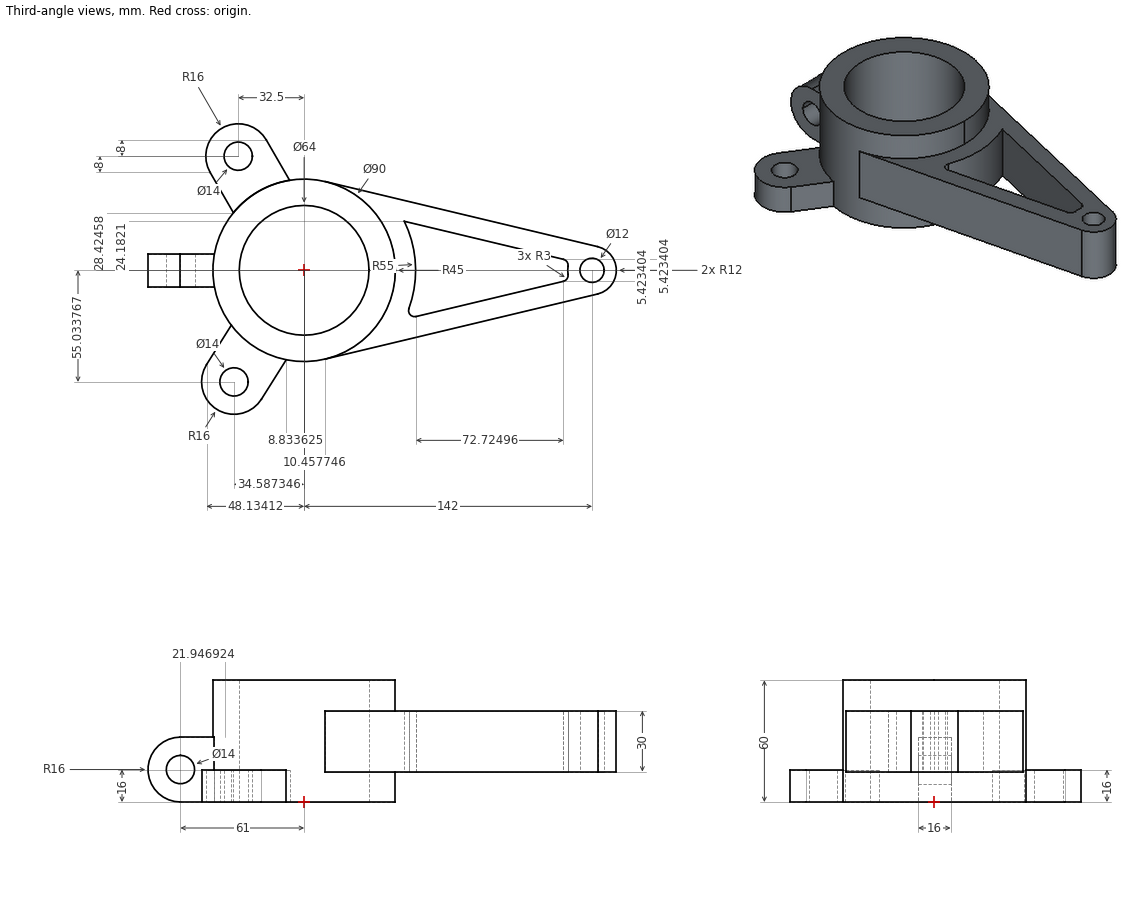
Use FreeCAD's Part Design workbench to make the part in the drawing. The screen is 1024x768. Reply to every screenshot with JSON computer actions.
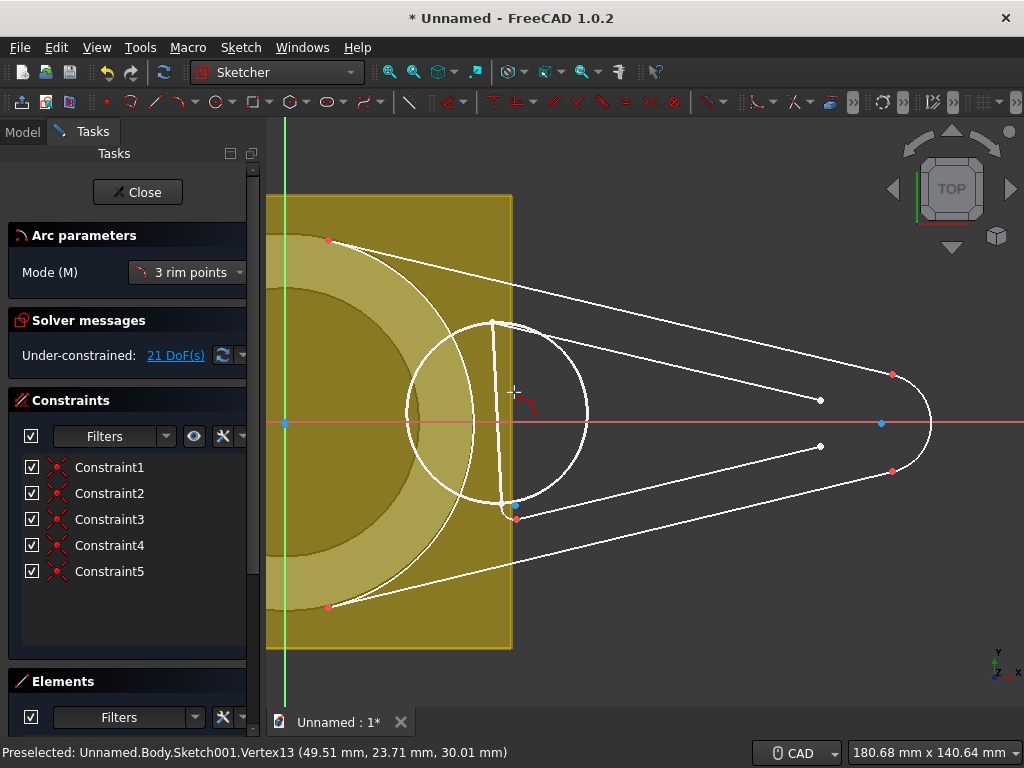
{"action": "left_click", "coordinate": [514, 392]}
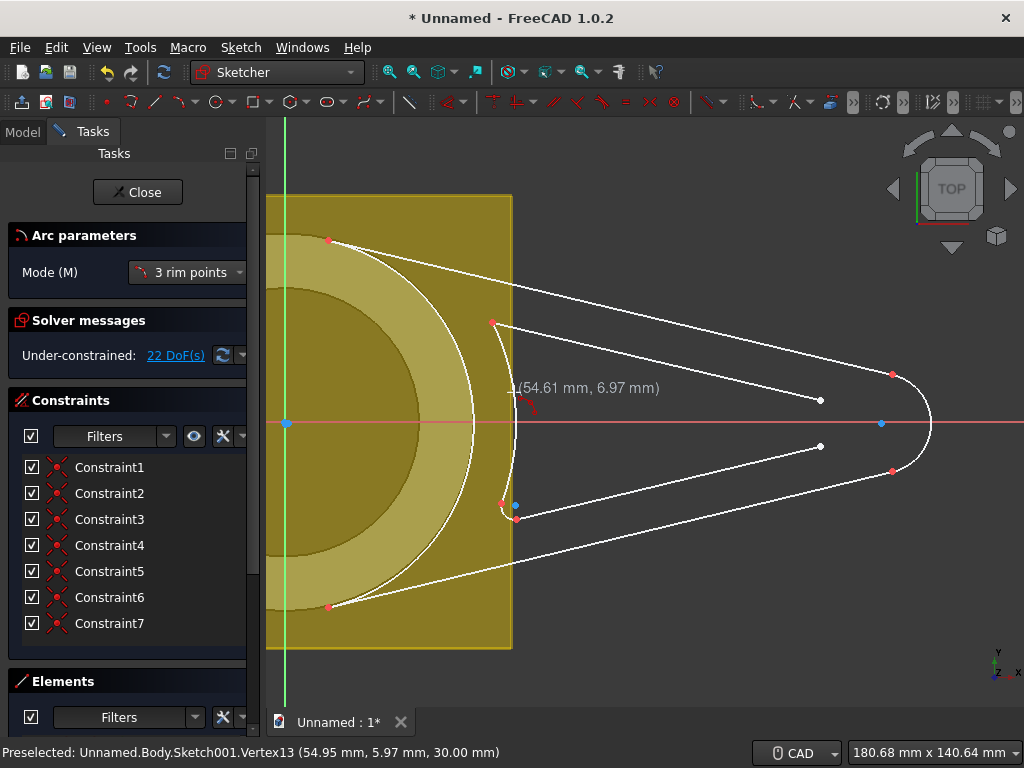
{"action": "left_click", "coordinate": [821, 400]}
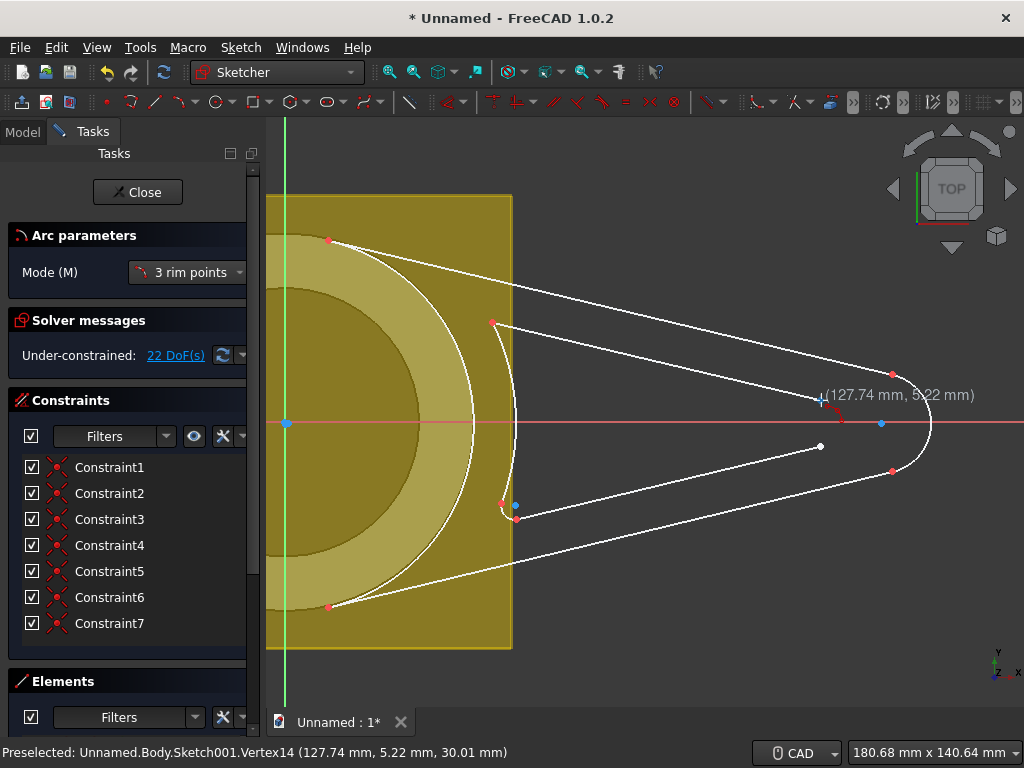
{"action": "scroll", "coordinate": [831, 414], "scroll_direction": "up", "scroll_amount": 4}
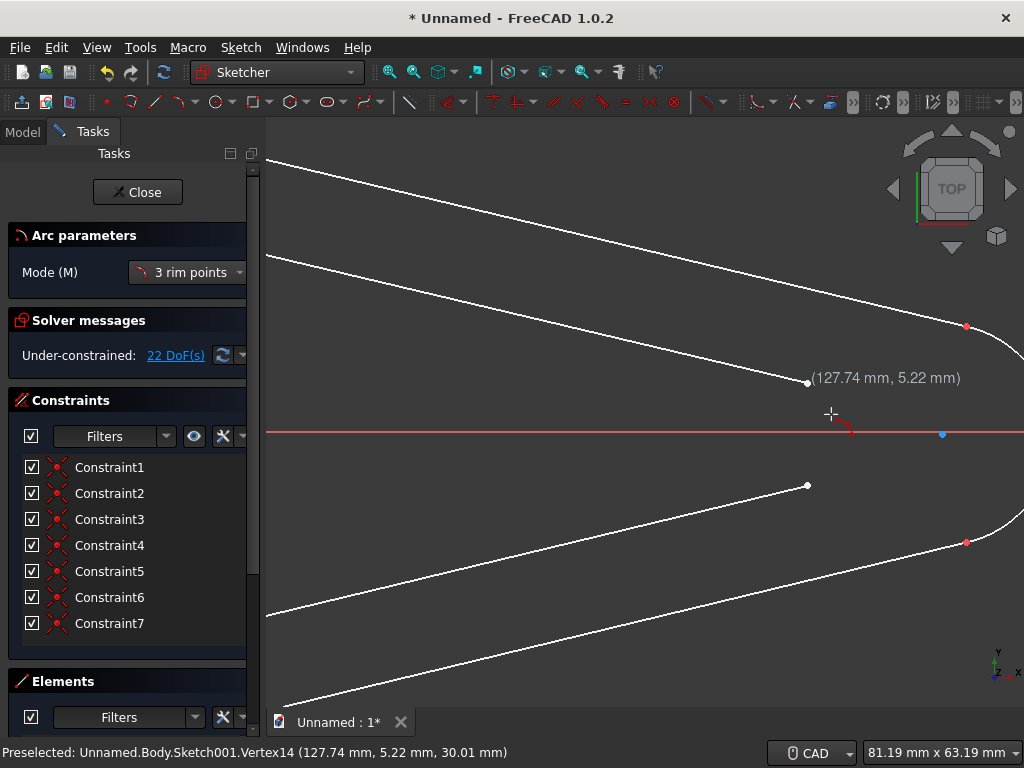
{"action": "left_click", "coordinate": [830, 413]}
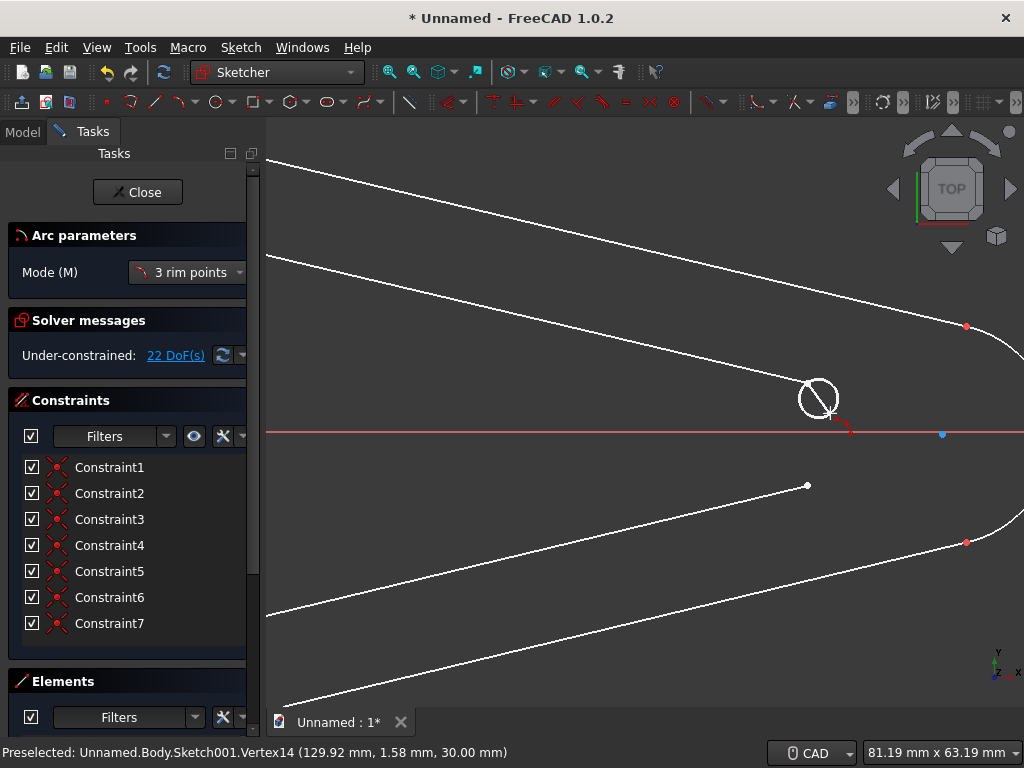
{"action": "scroll", "coordinate": [826, 393], "scroll_direction": "up", "scroll_amount": 4}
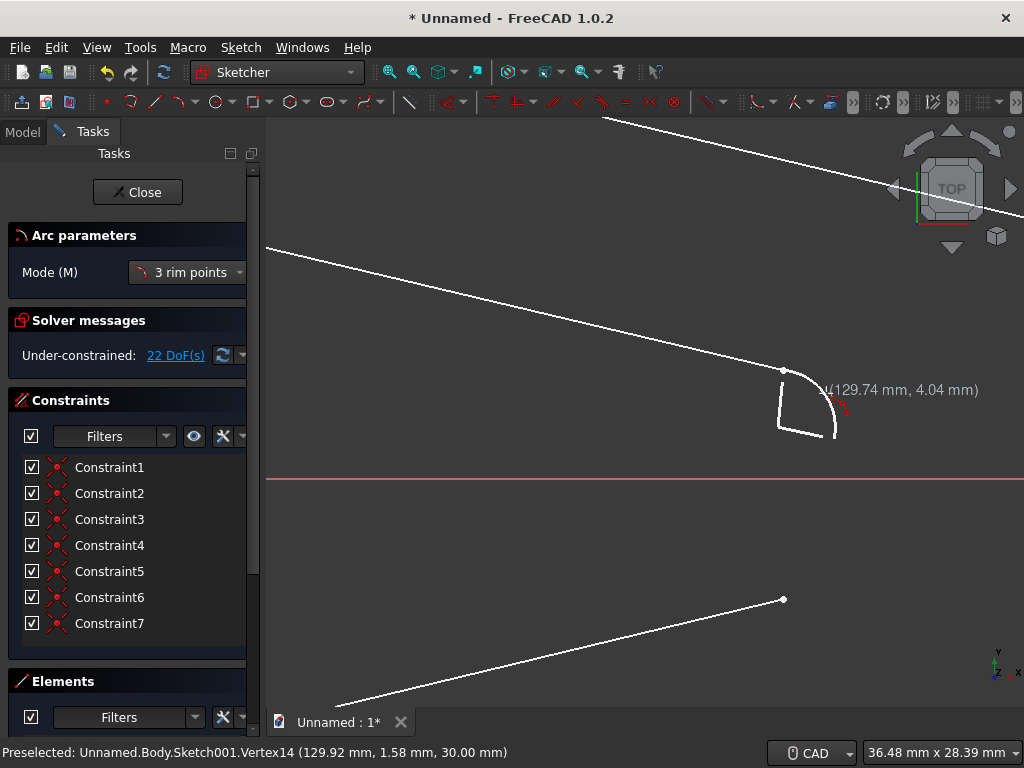
{"action": "left_click", "coordinate": [825, 392]}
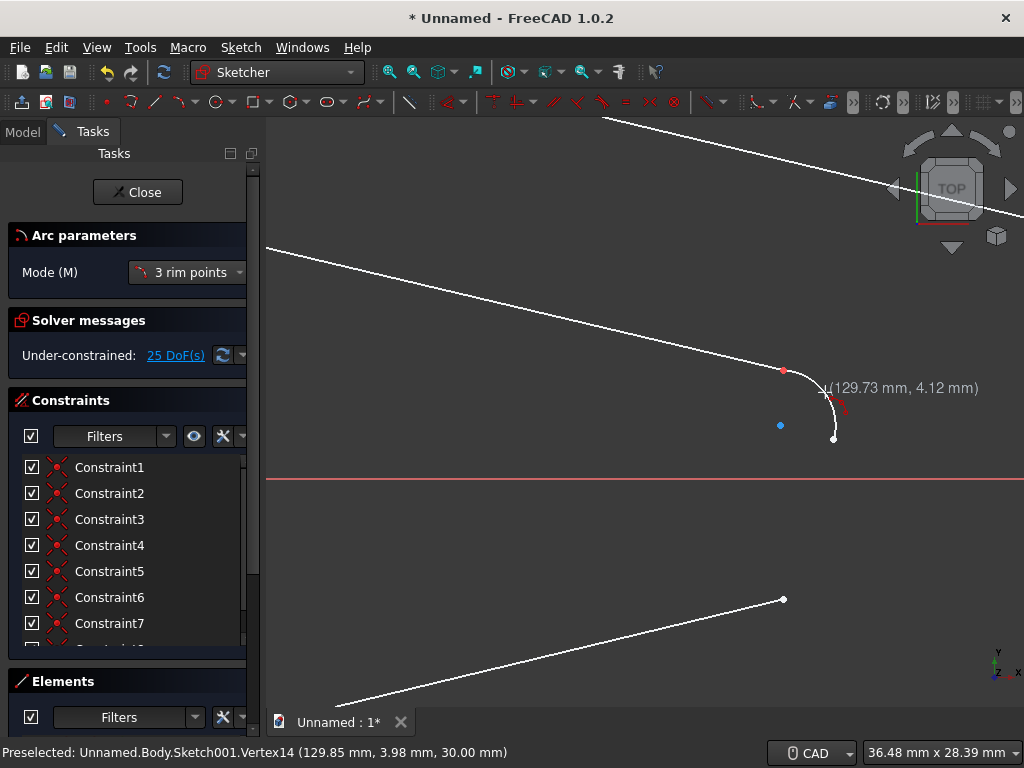
{"action": "left_click", "coordinate": [834, 439]}
{"action": "left_click", "coordinate": [834, 520]}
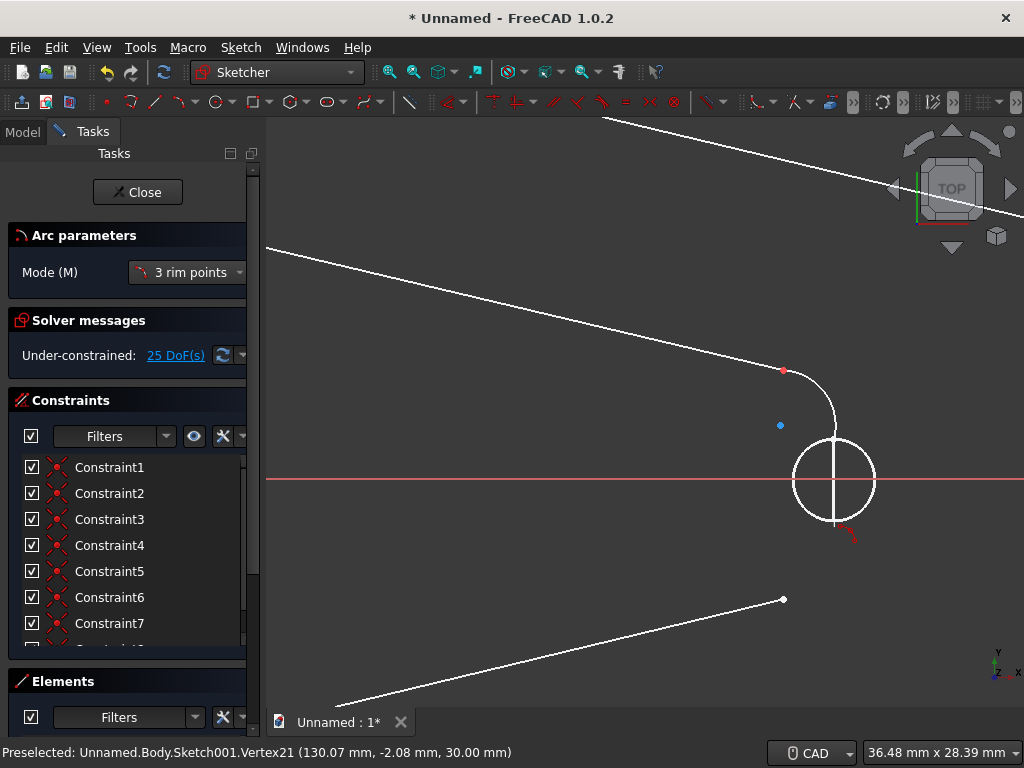
{"action": "scroll", "coordinate": [831, 470], "scroll_direction": "up", "scroll_amount": 8}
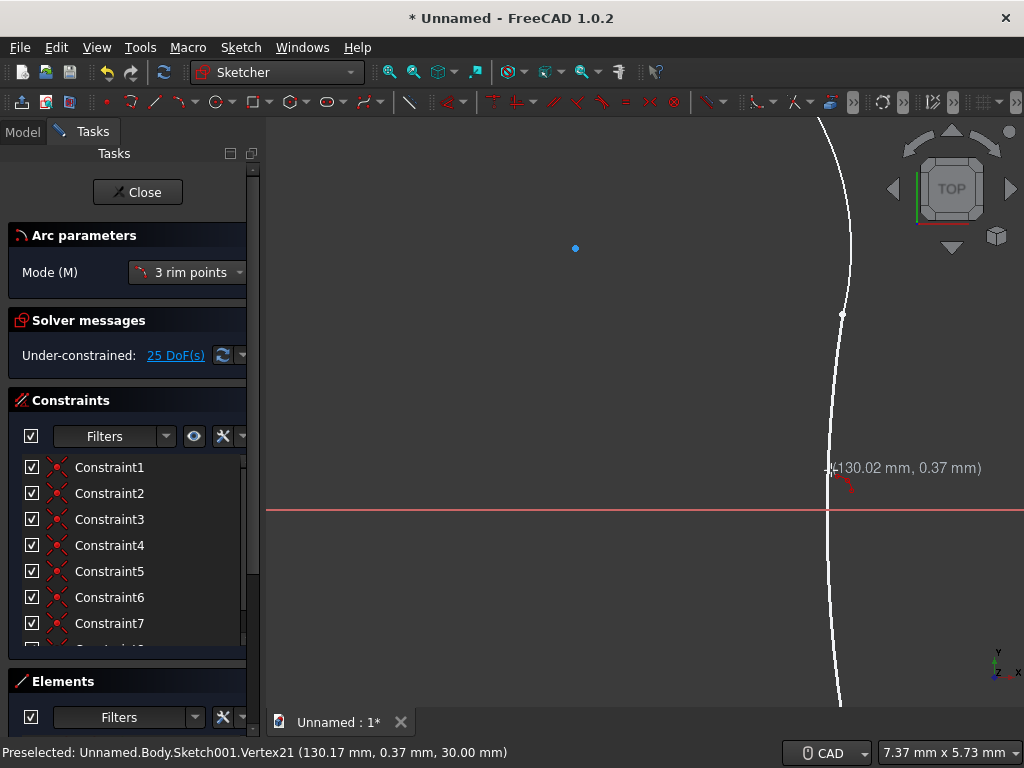
{"action": "left_click", "coordinate": [826, 469]}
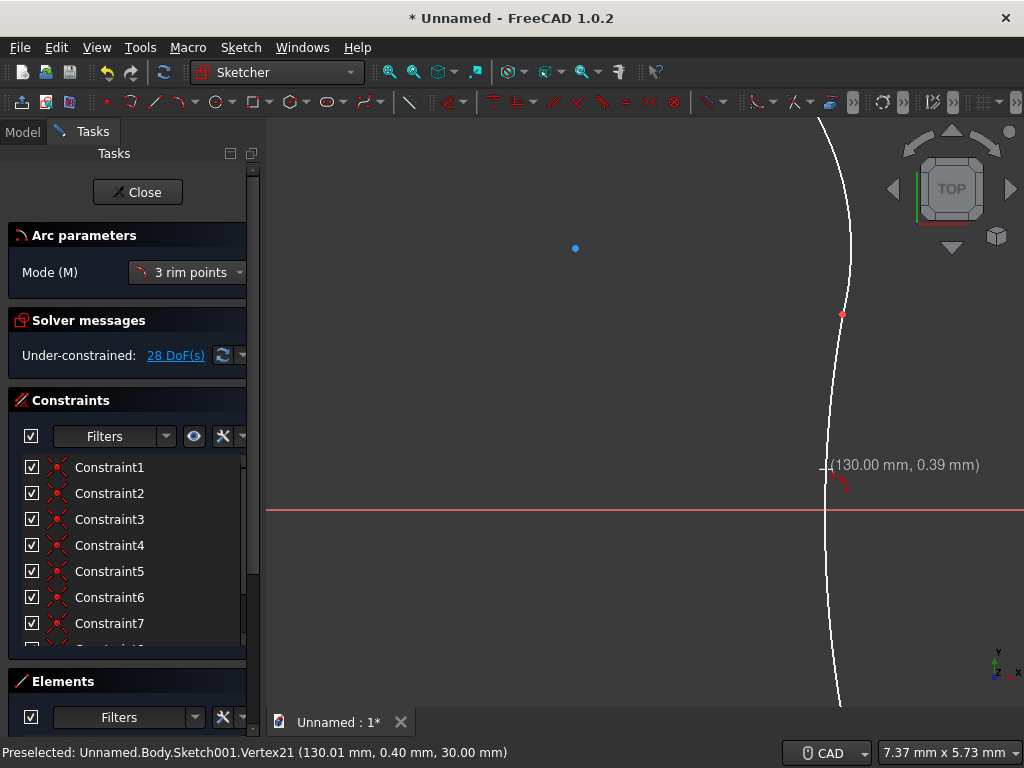
{"action": "scroll", "coordinate": [723, 409], "scroll_direction": "down", "scroll_amount": 18}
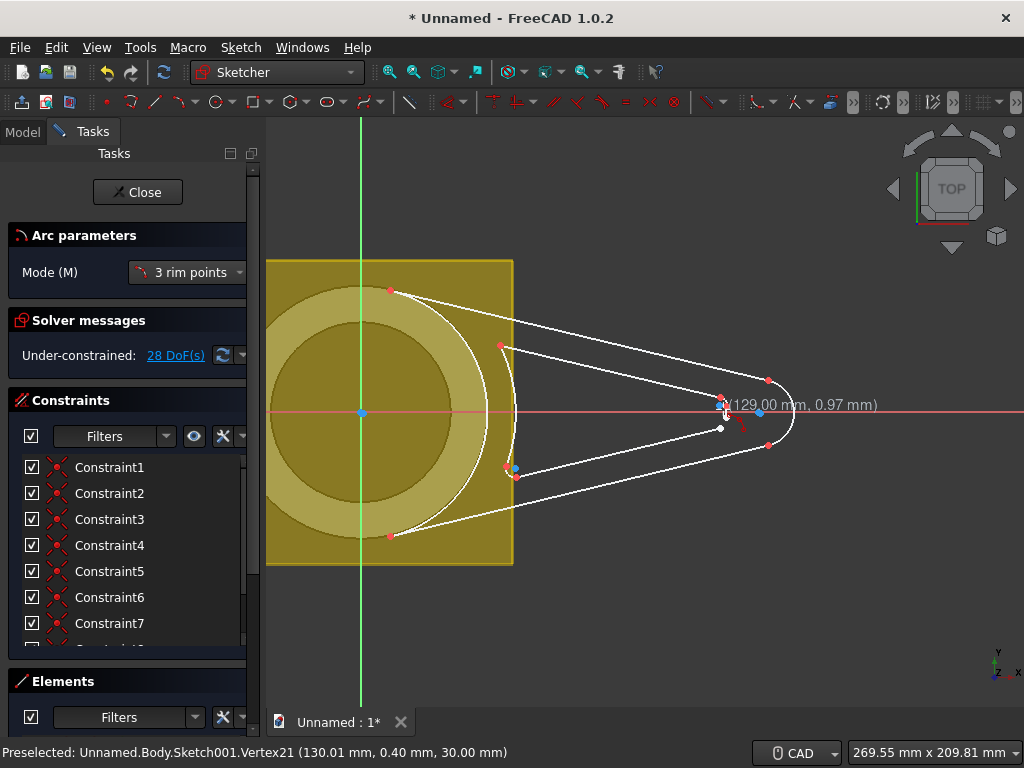
{"action": "scroll", "coordinate": [727, 418], "scroll_direction": "up", "scroll_amount": 6}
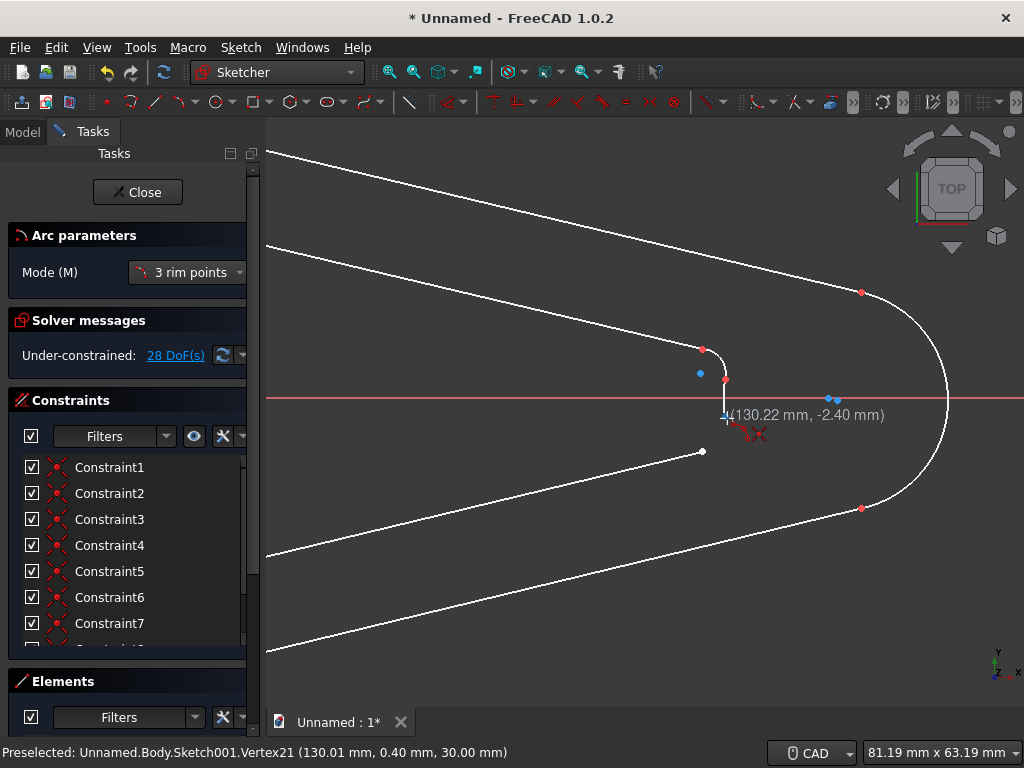
{"action": "left_click", "coordinate": [725, 417]}
{"action": "left_click", "coordinate": [702, 452]}